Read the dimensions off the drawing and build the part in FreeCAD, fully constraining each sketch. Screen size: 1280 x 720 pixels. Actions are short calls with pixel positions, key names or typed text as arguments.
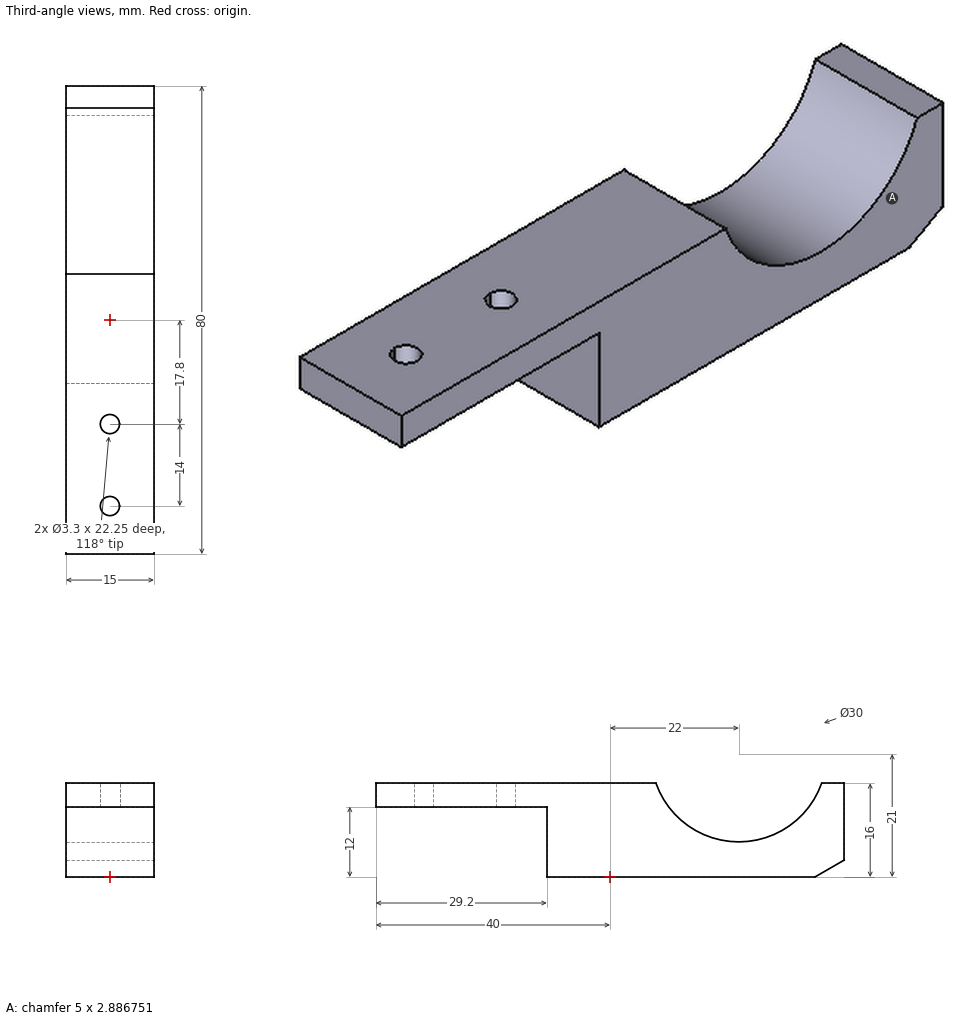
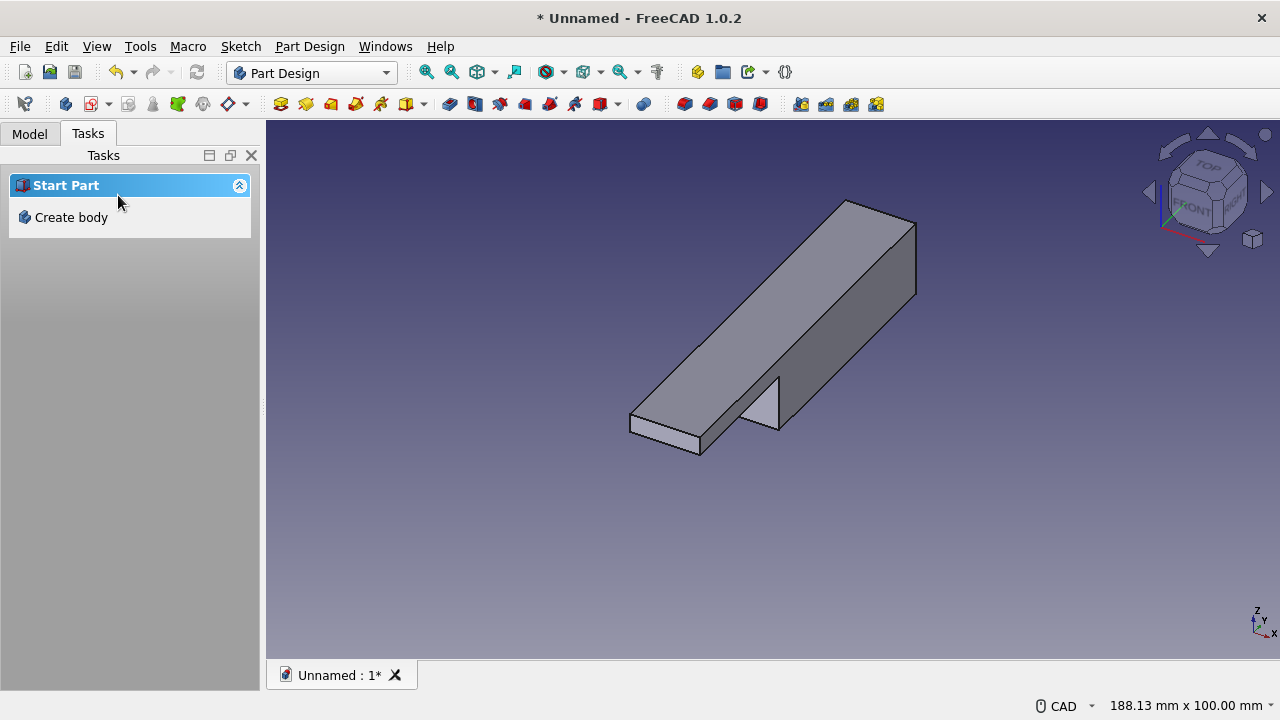
key(5)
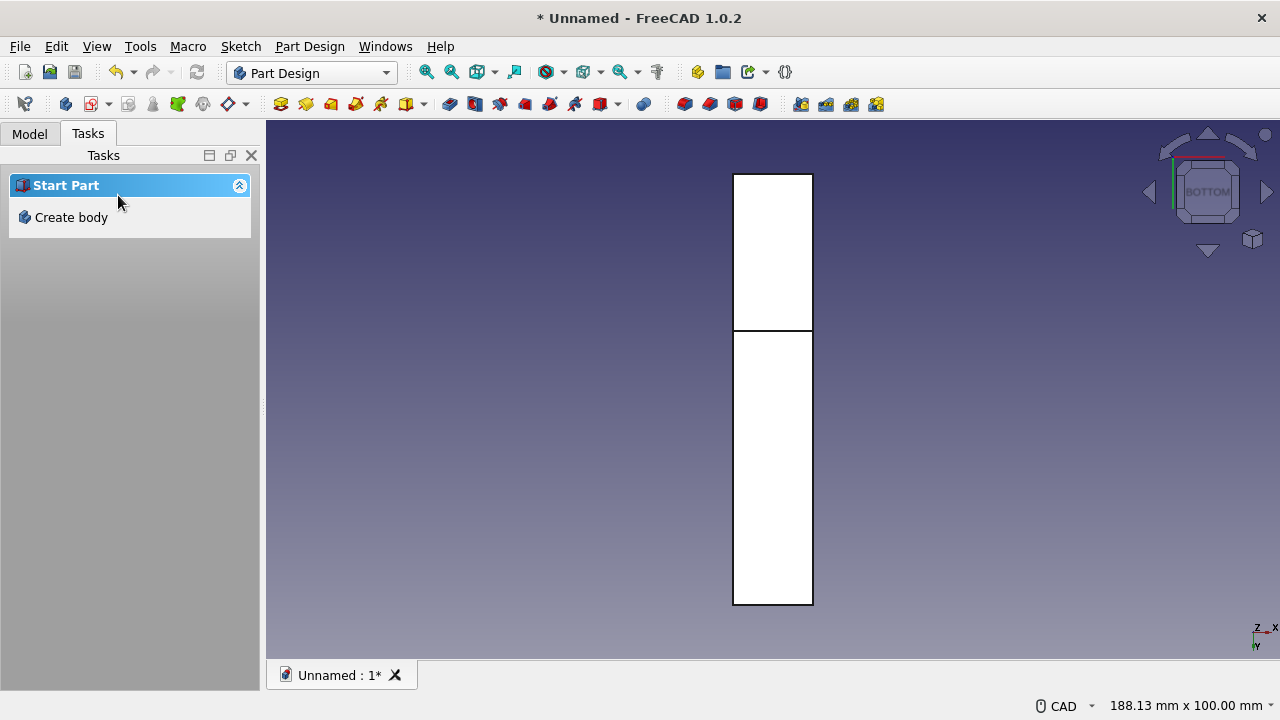
click(773, 274)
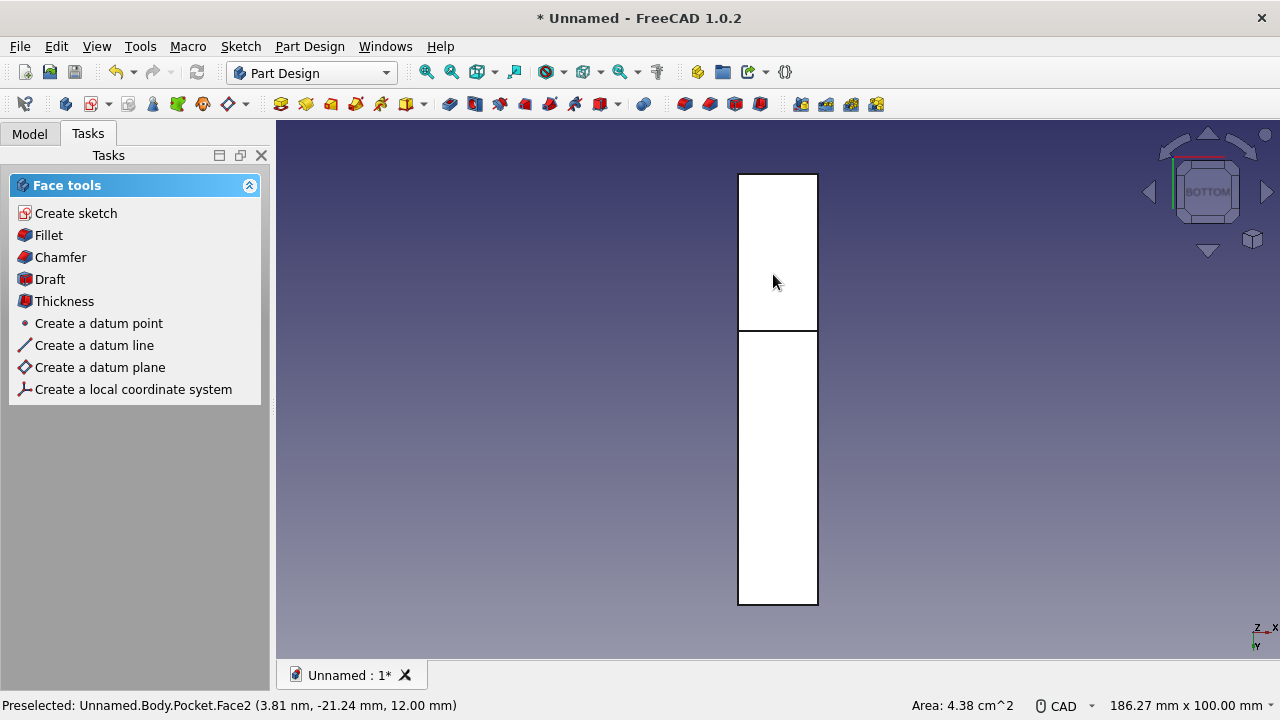
click(90, 104)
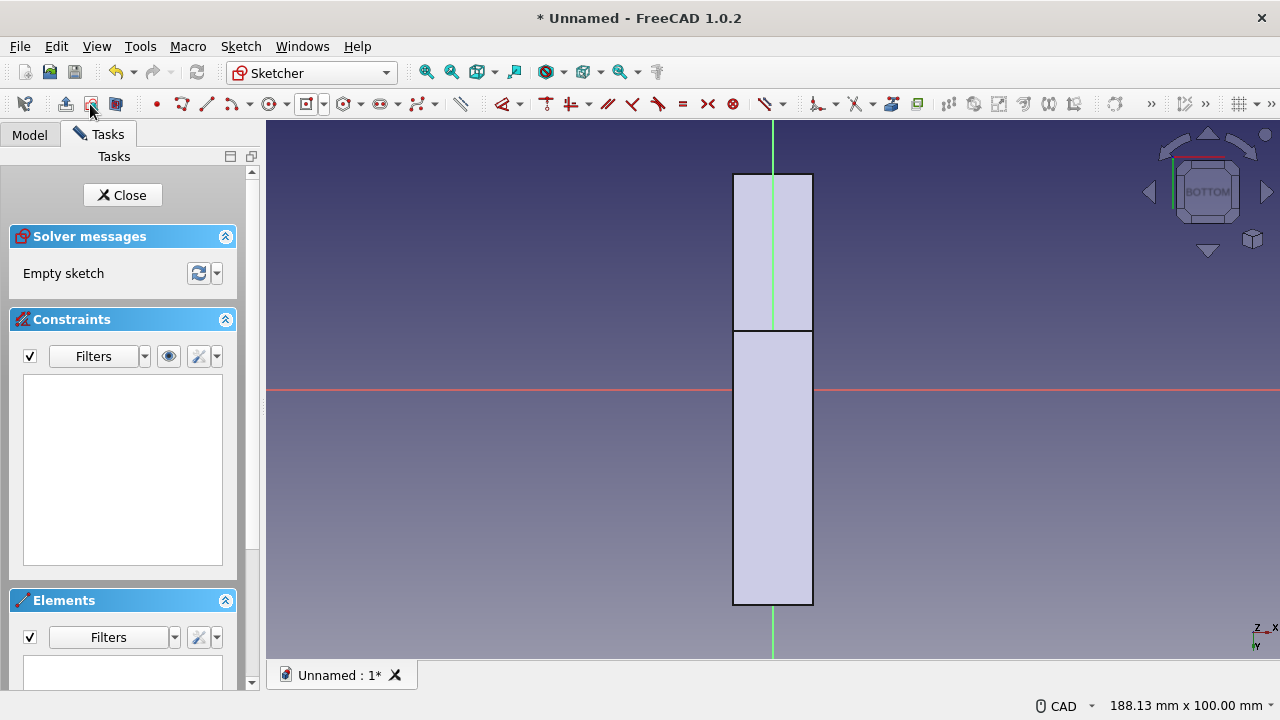
key(q)
key(s)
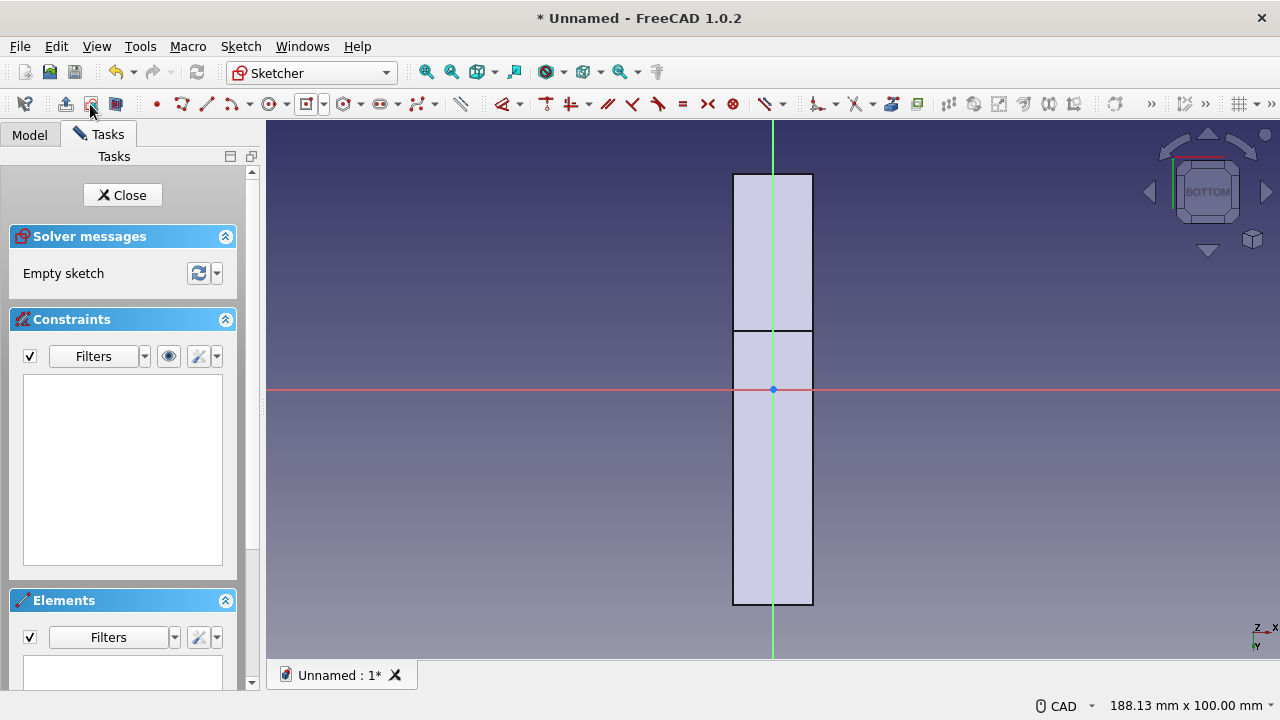
scroll(856, 190, up, 3)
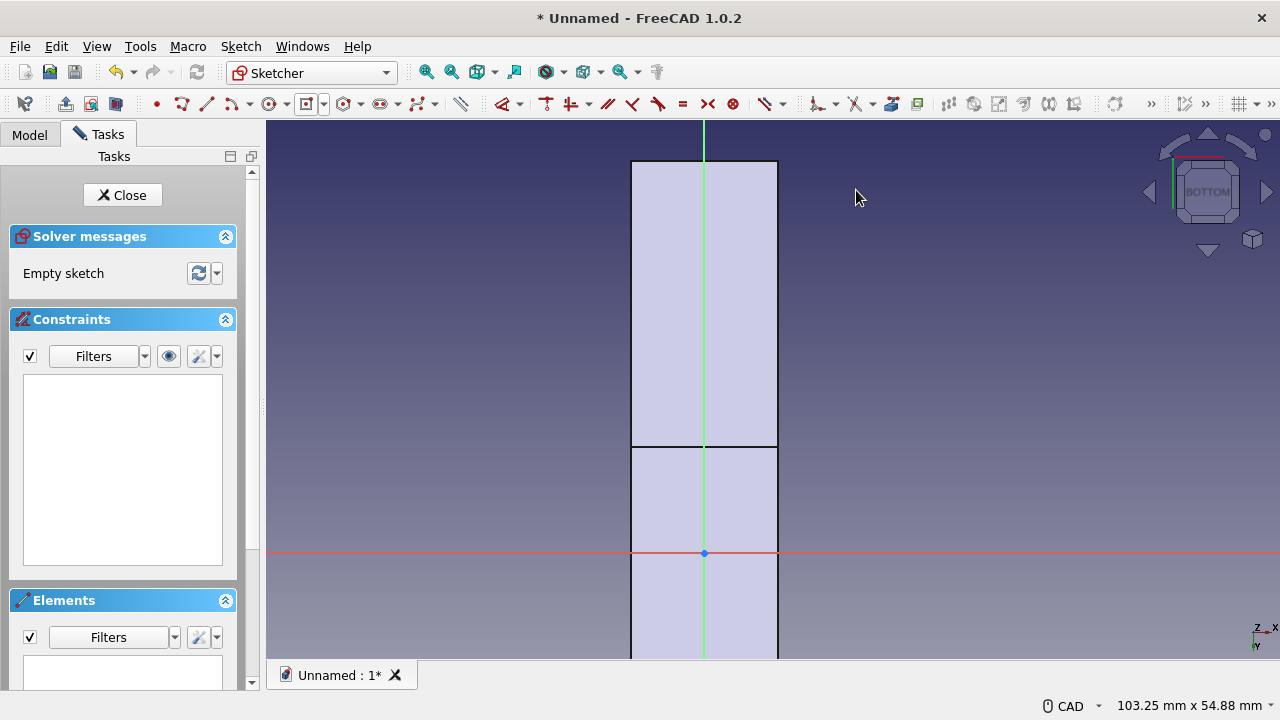
click(268, 104)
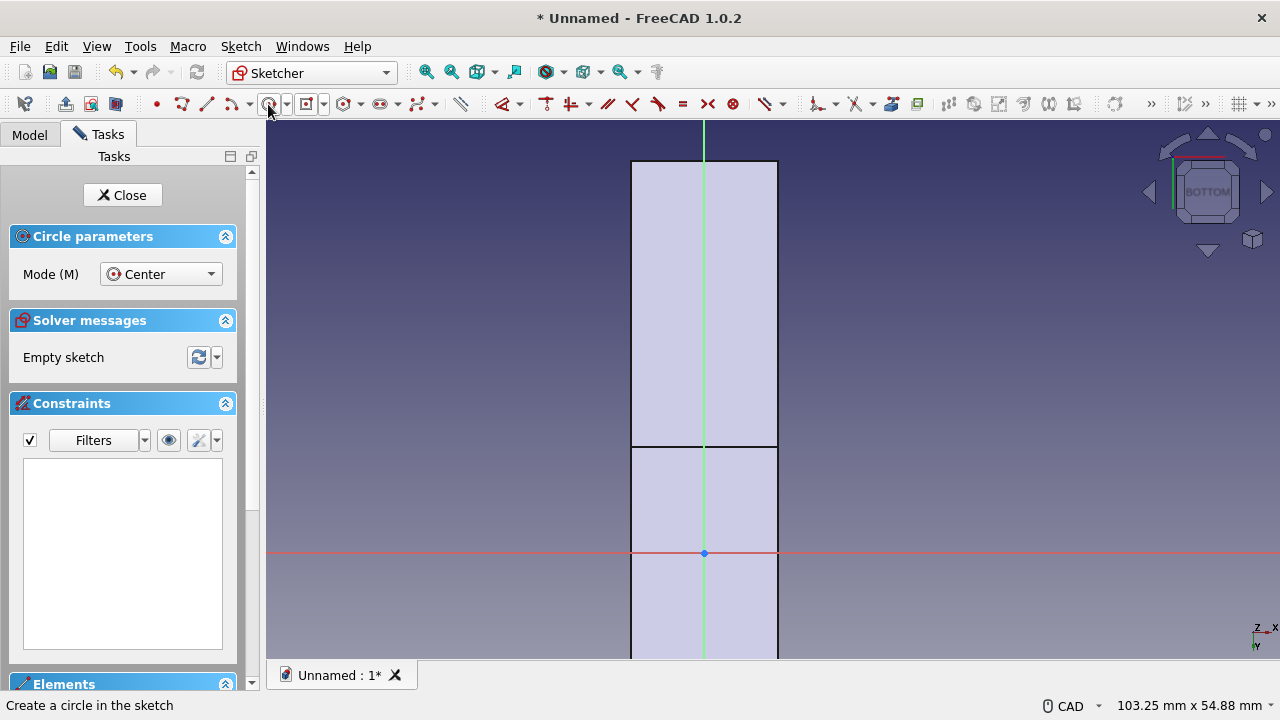
scroll(704, 379, up, 2)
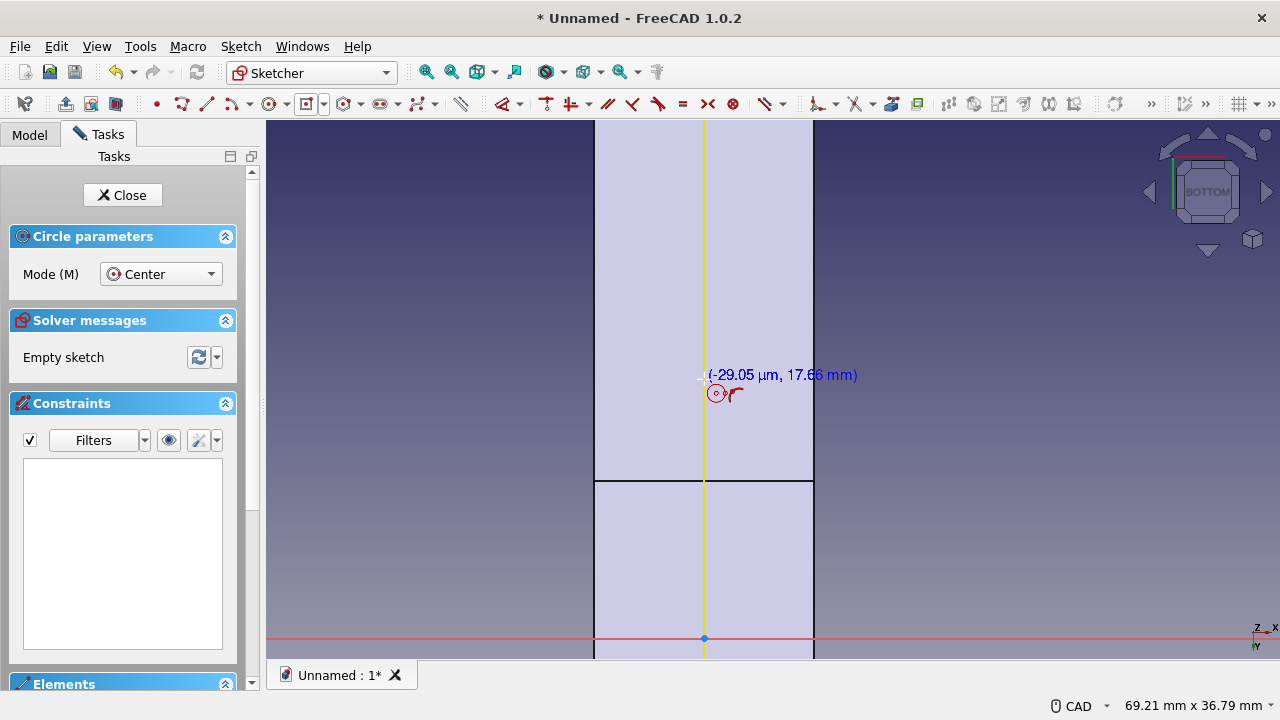
click(704, 378)
click(721, 361)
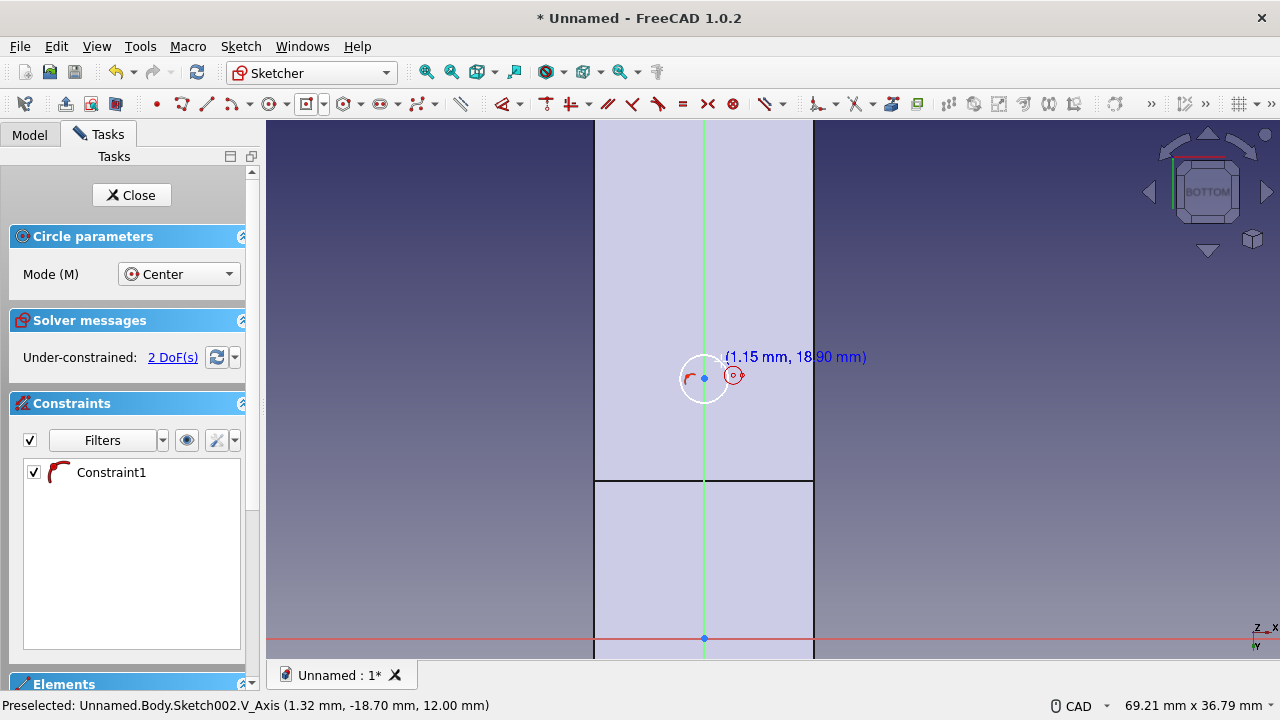
click(704, 173)
click(721, 156)
key(Escape)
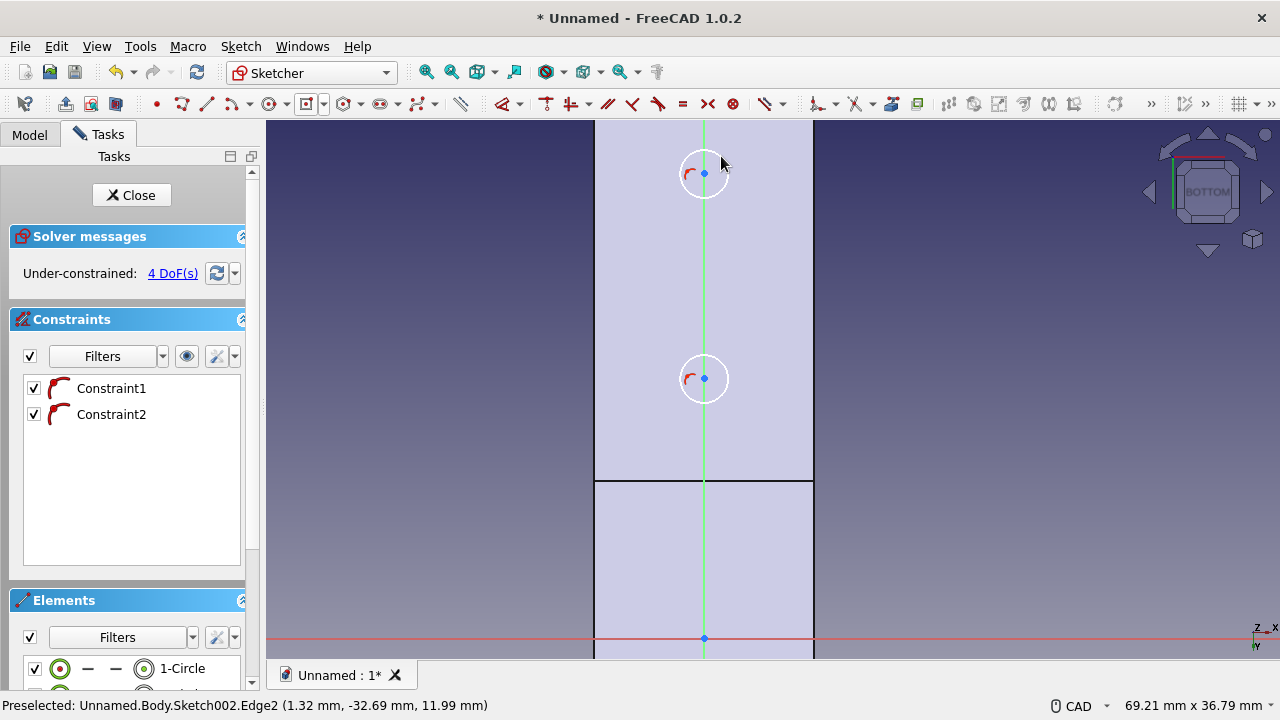
click(721, 362)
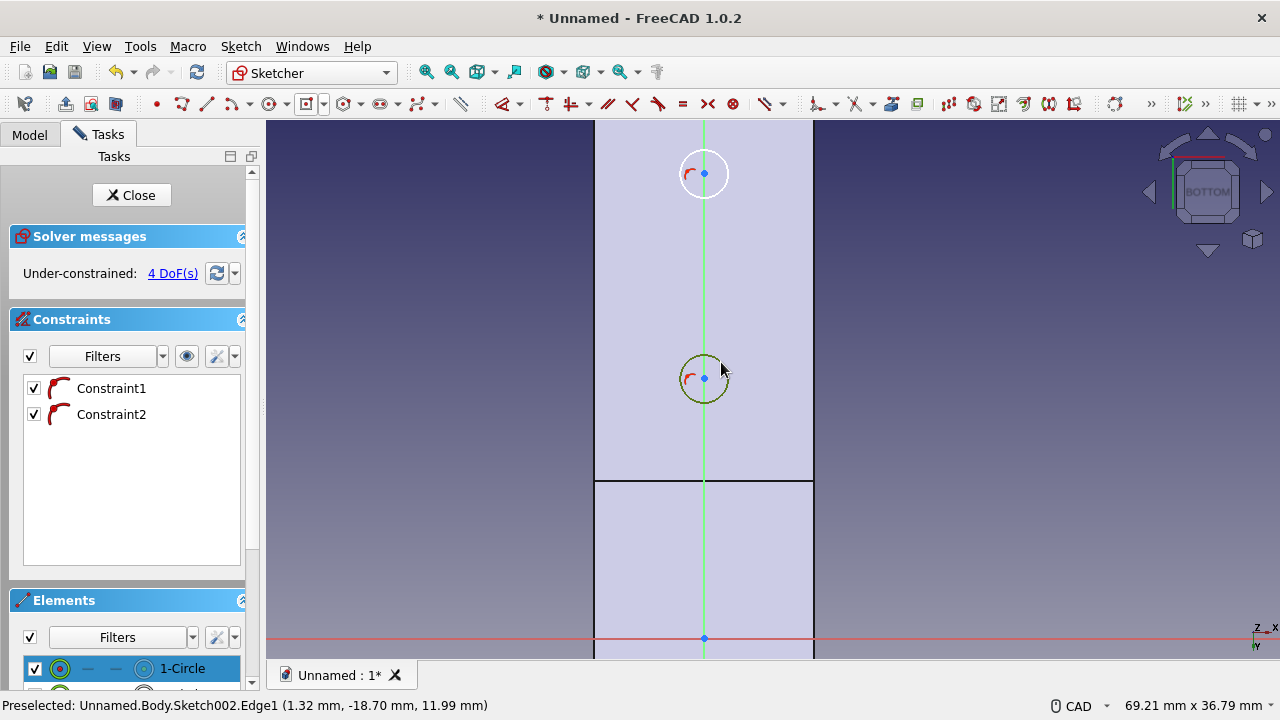
click(721, 157)